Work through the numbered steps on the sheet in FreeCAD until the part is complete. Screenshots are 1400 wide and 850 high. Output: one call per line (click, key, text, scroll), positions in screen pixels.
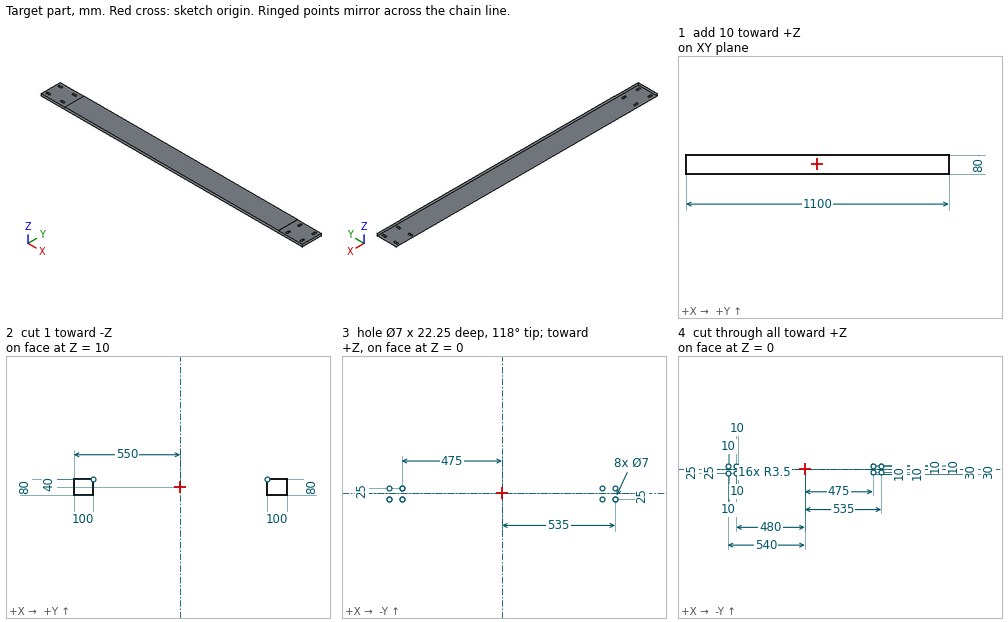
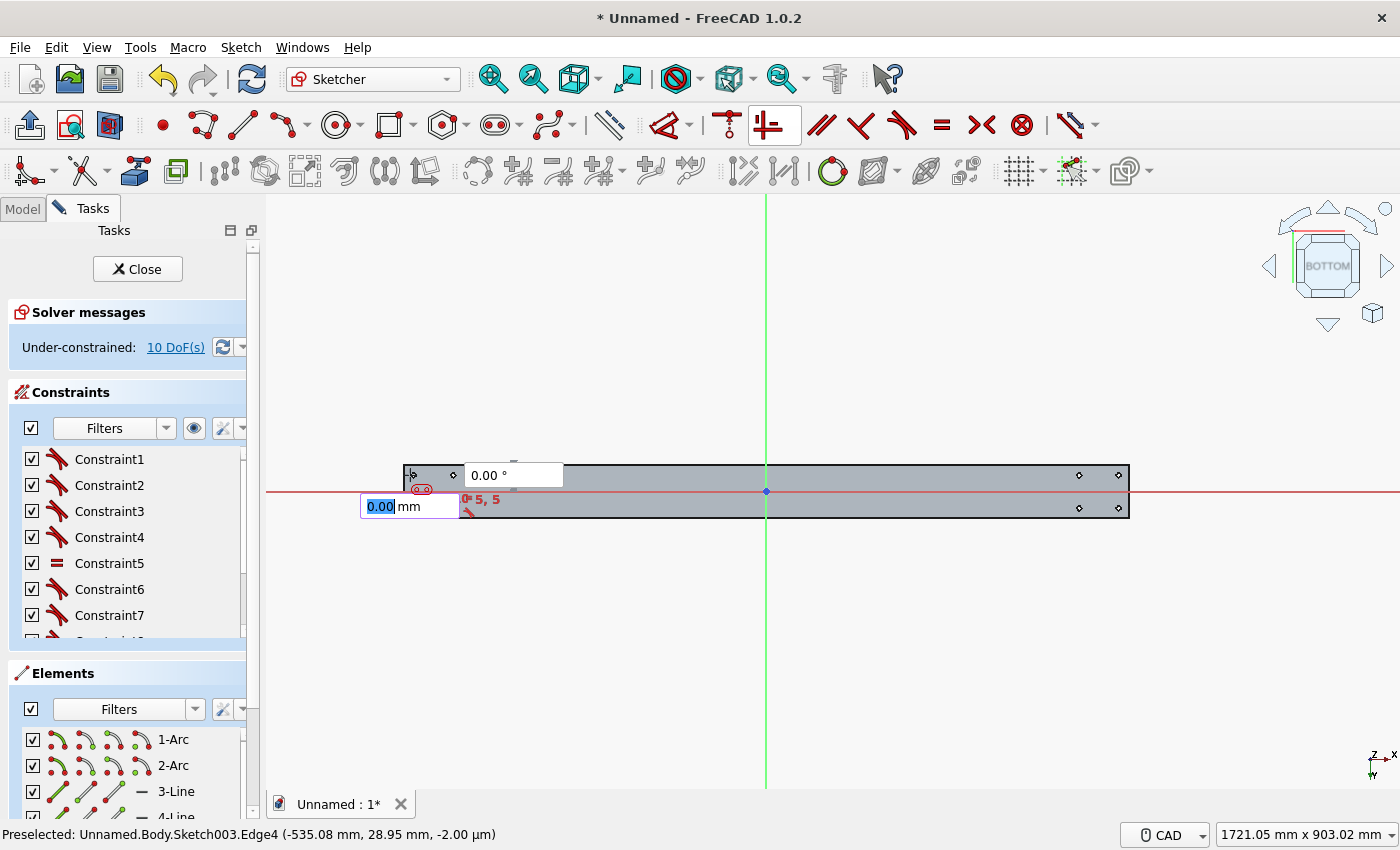
scroll(417, 475, up, 5)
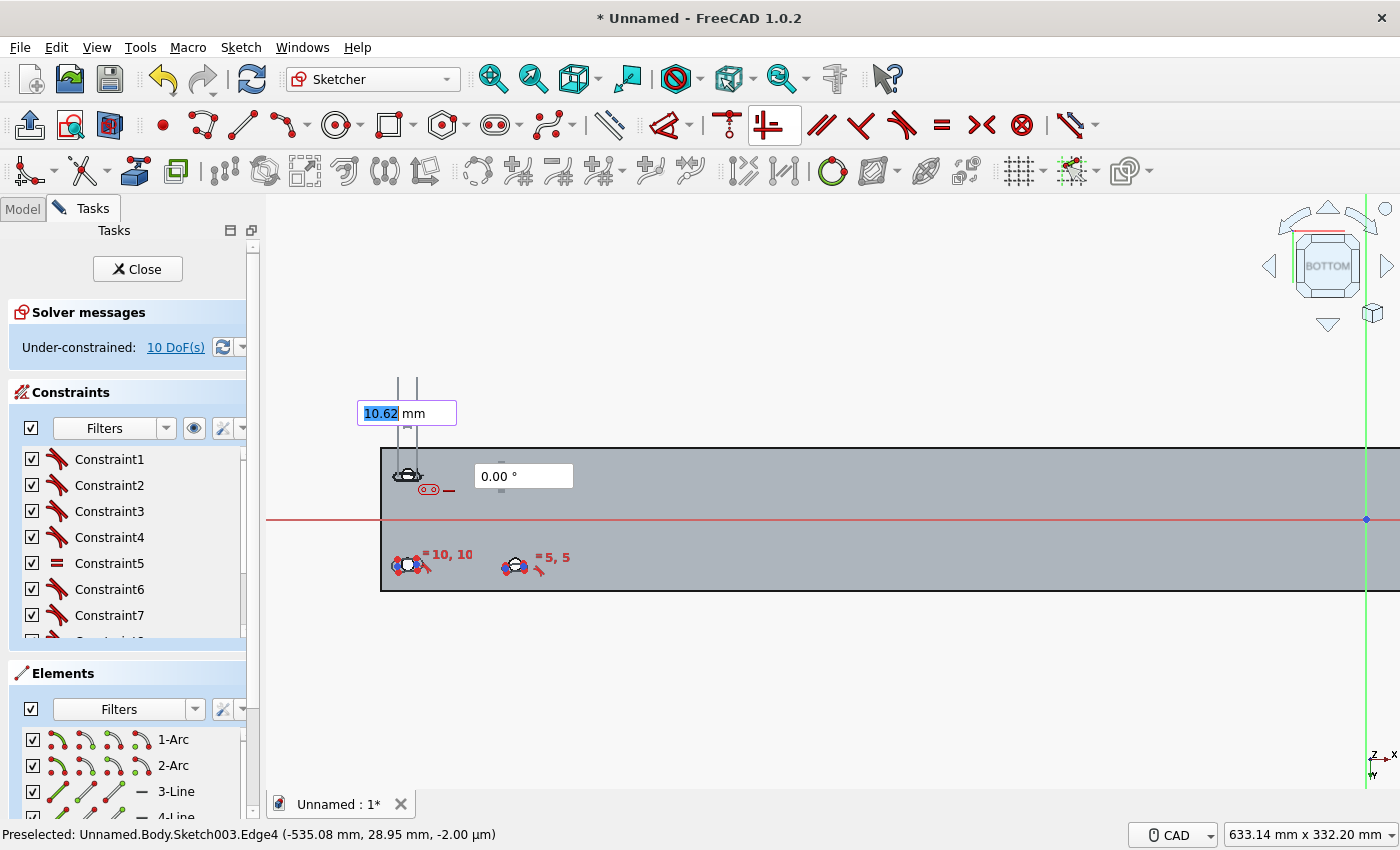
click(417, 474)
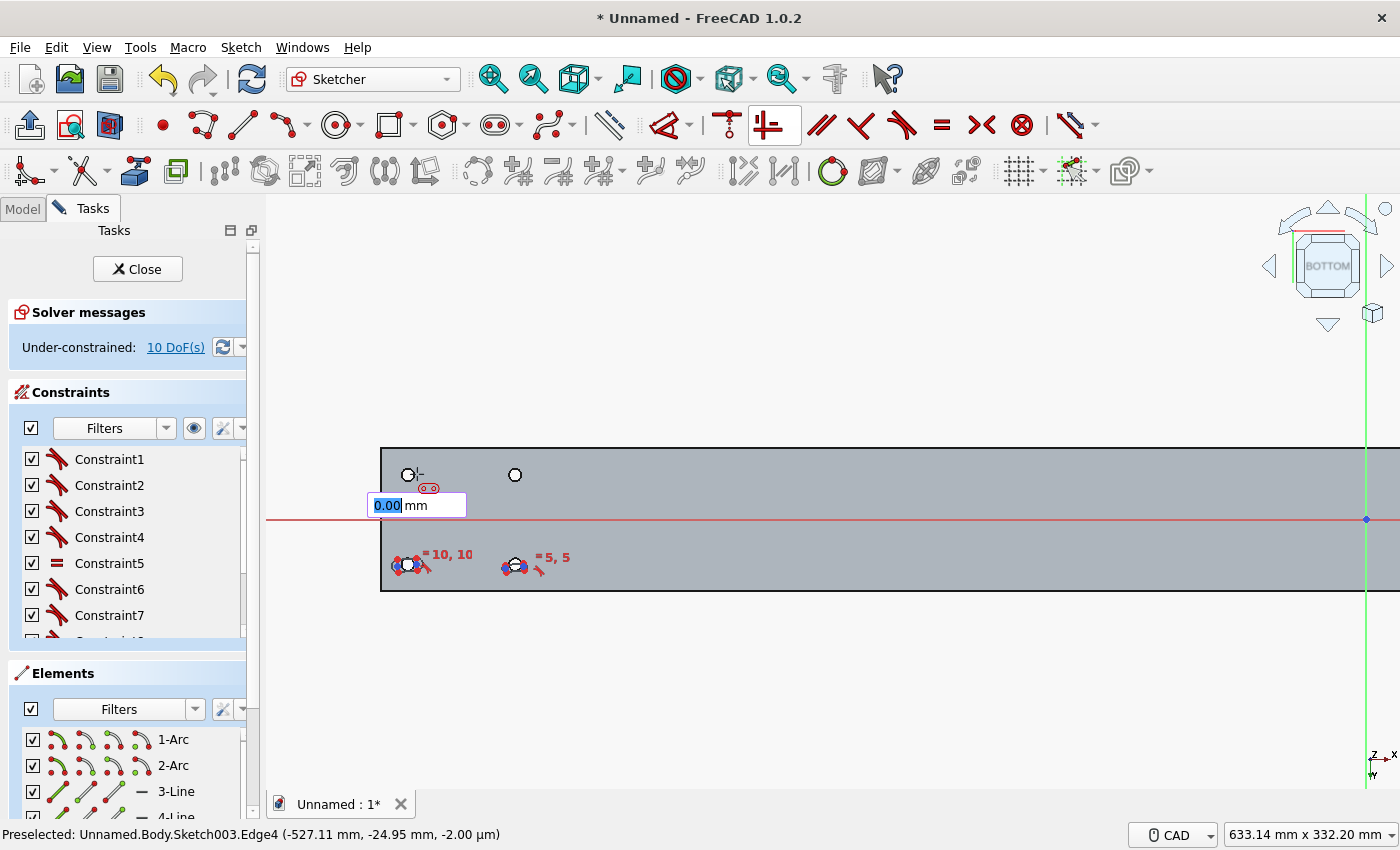
scroll(408, 481, up, 5)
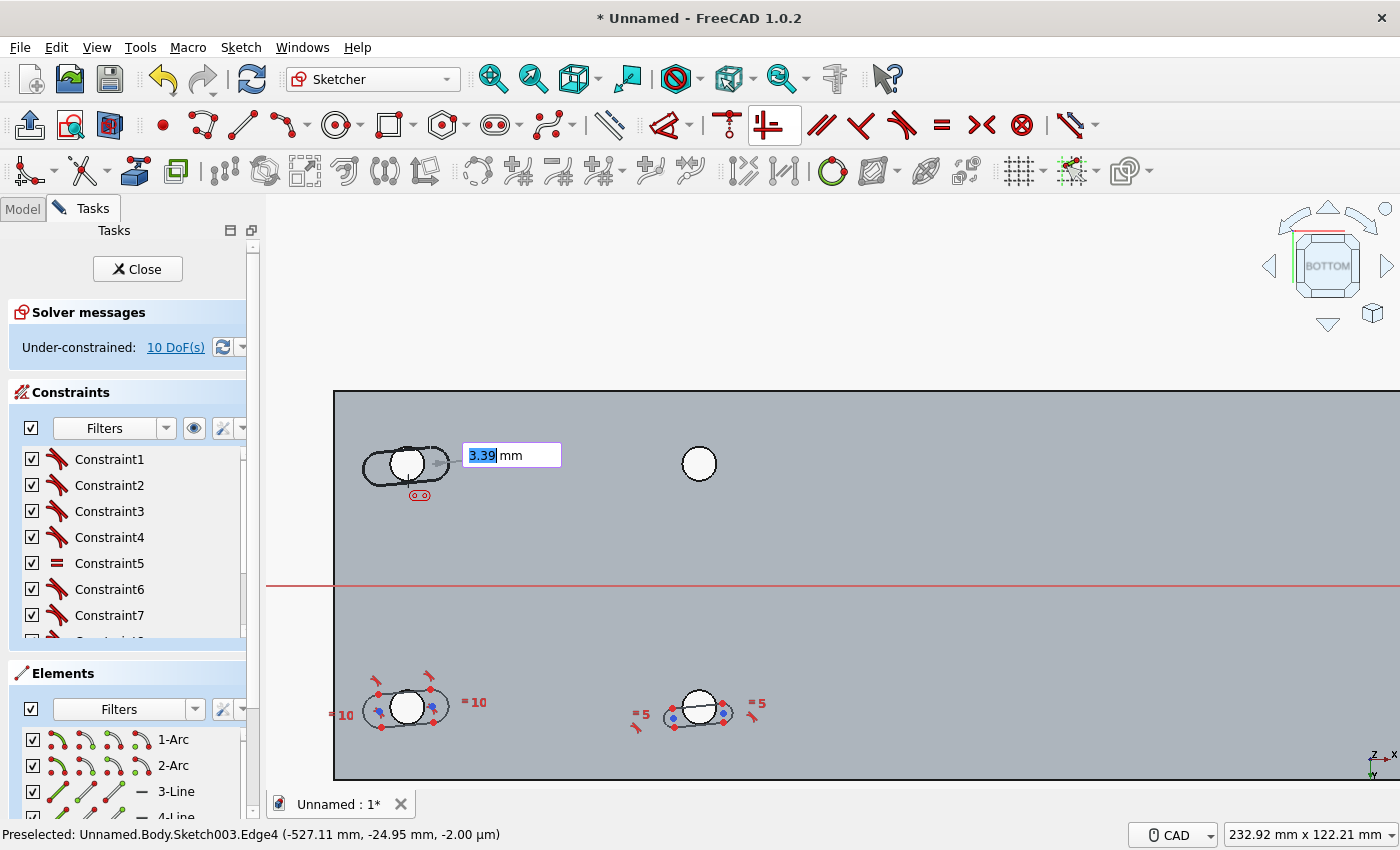
click(407, 481)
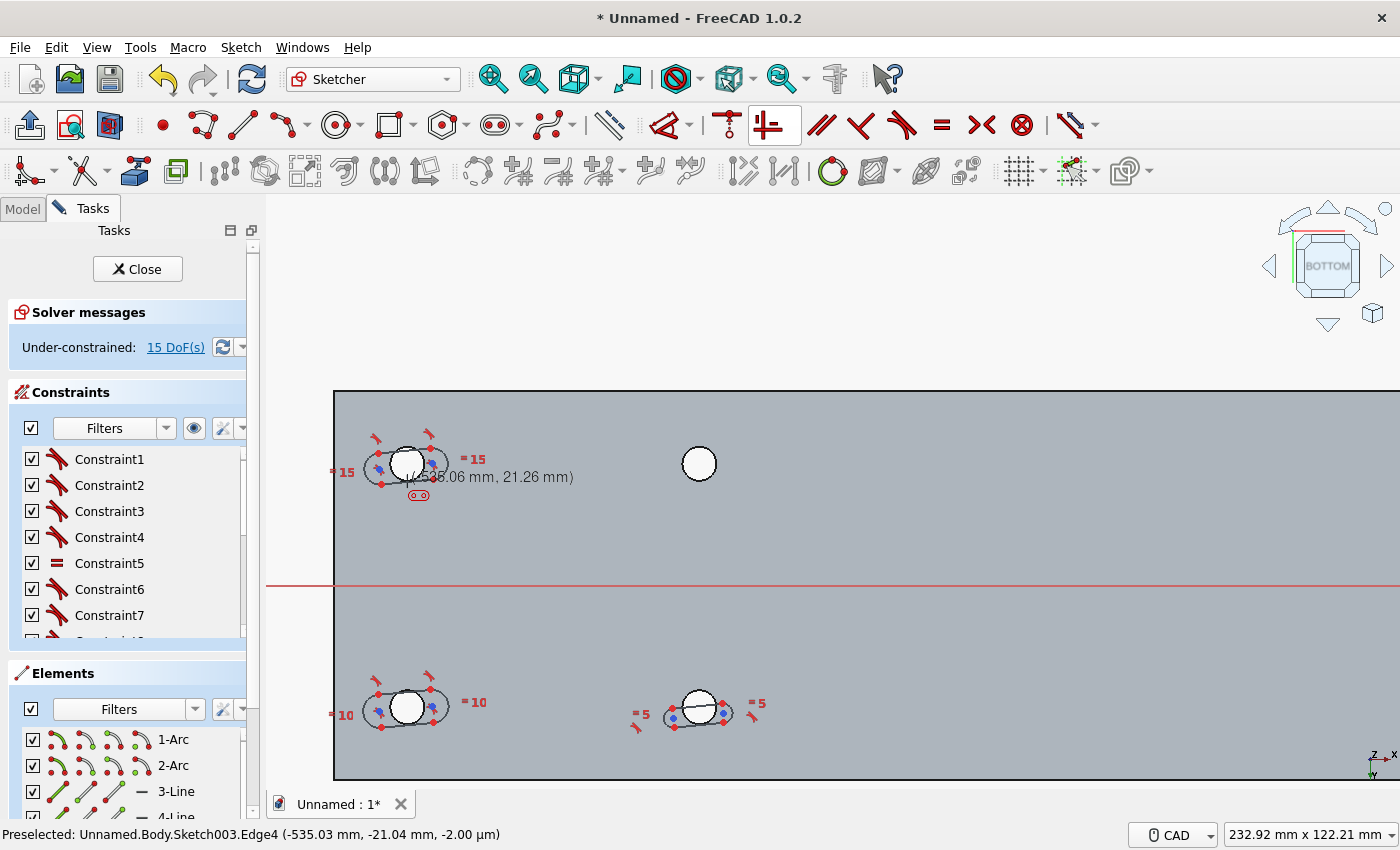
scroll(675, 464, up, 2)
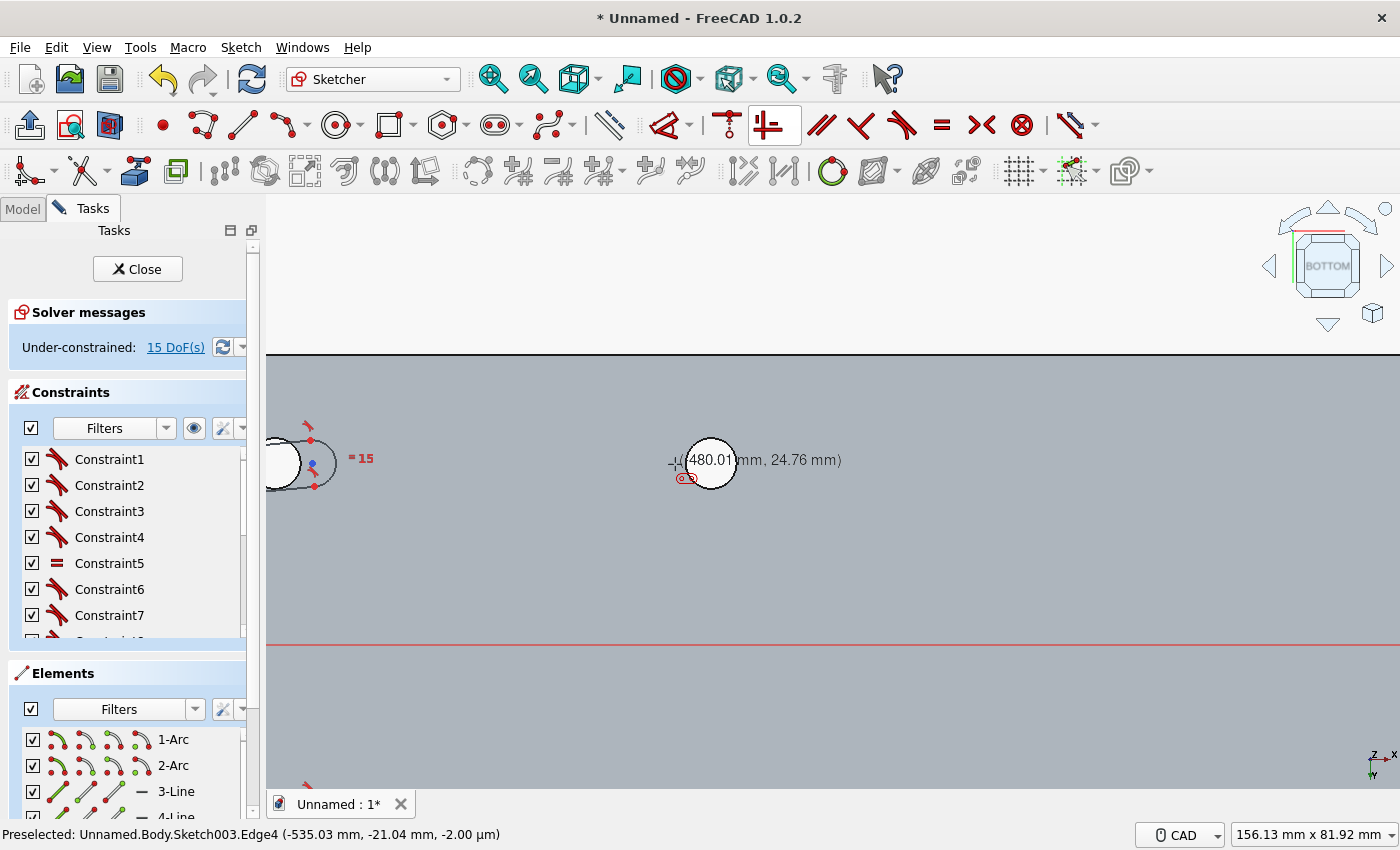
scroll(427, 476, down, 12)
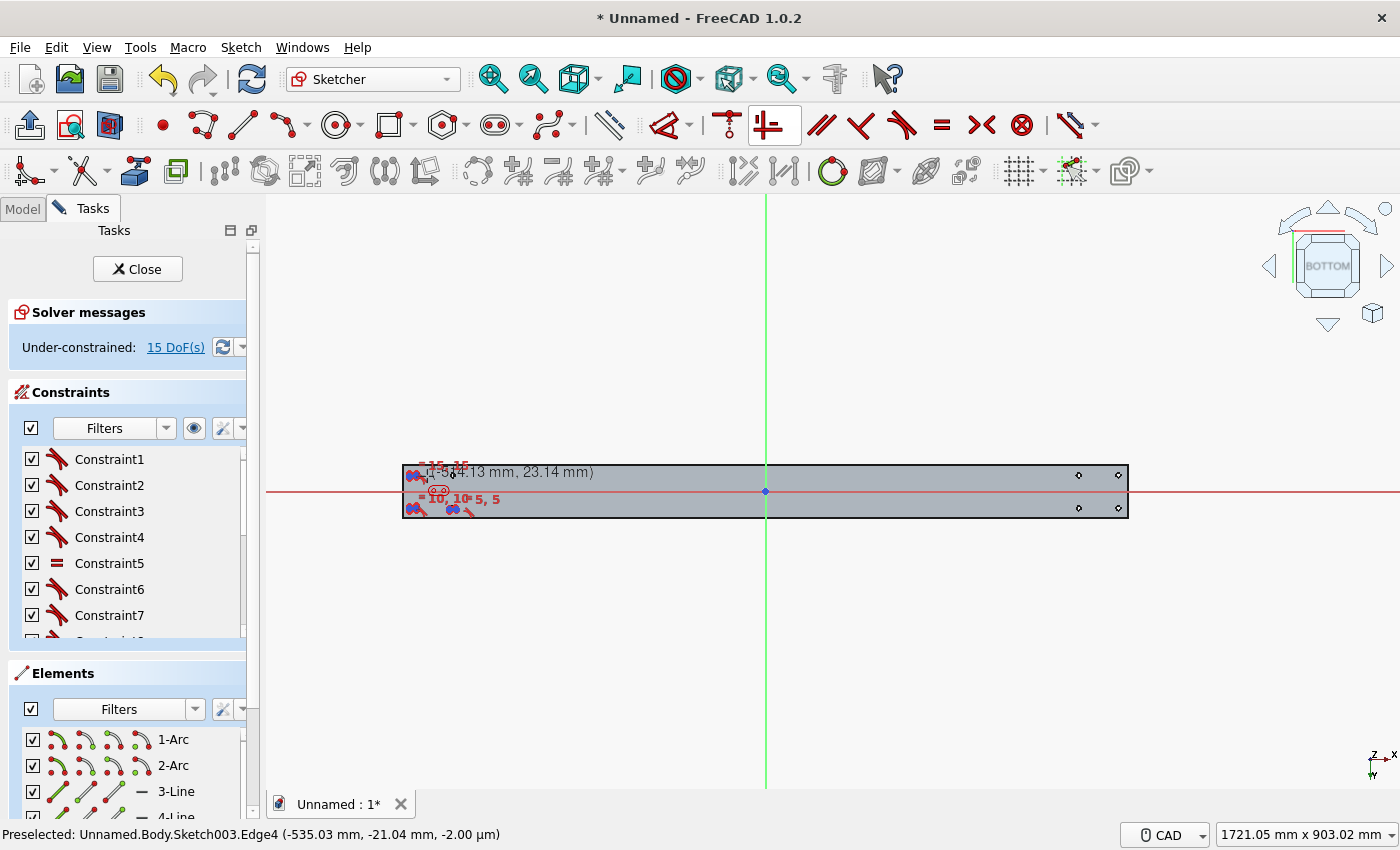
click(450, 475)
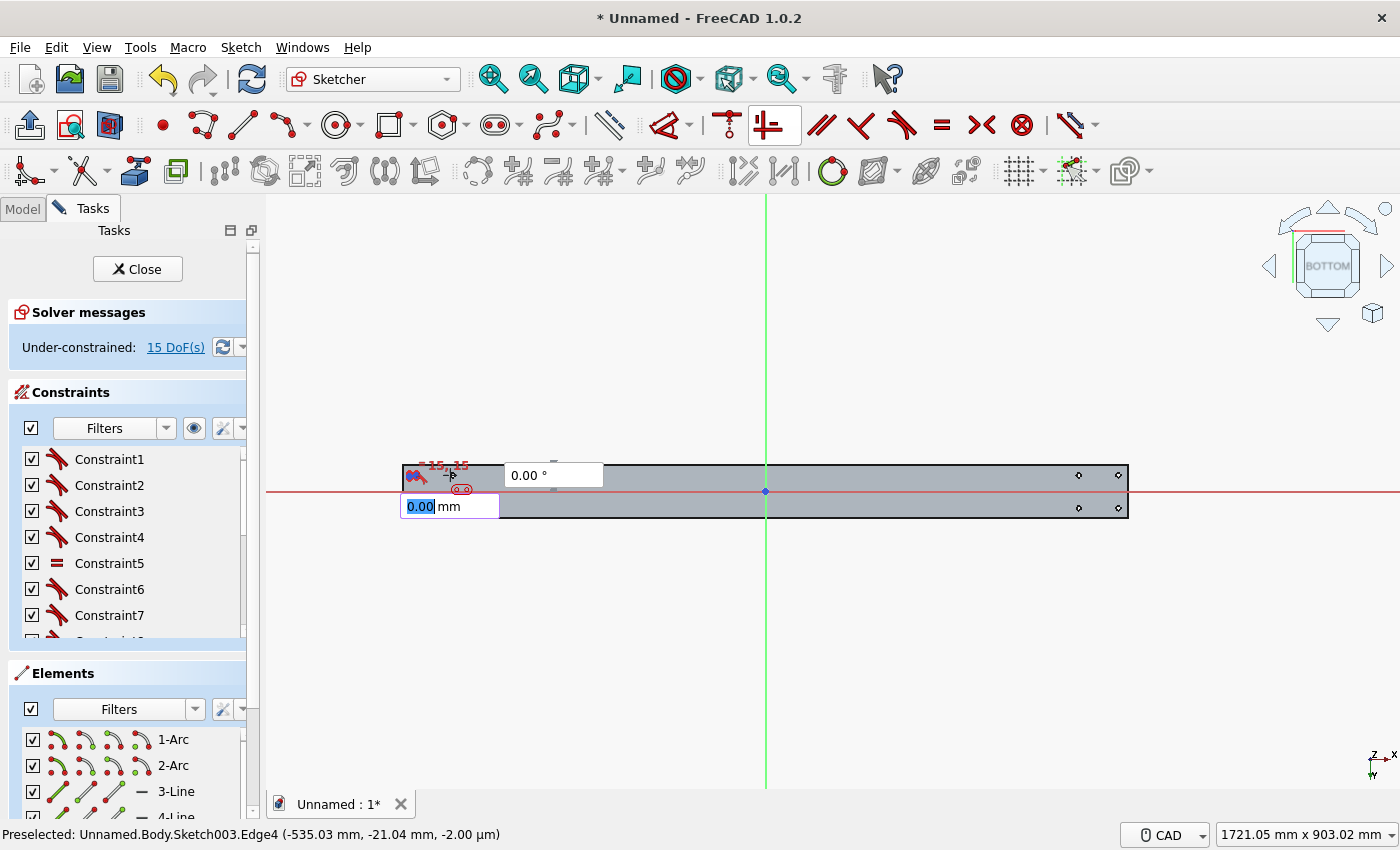
scroll(456, 475, up, 5)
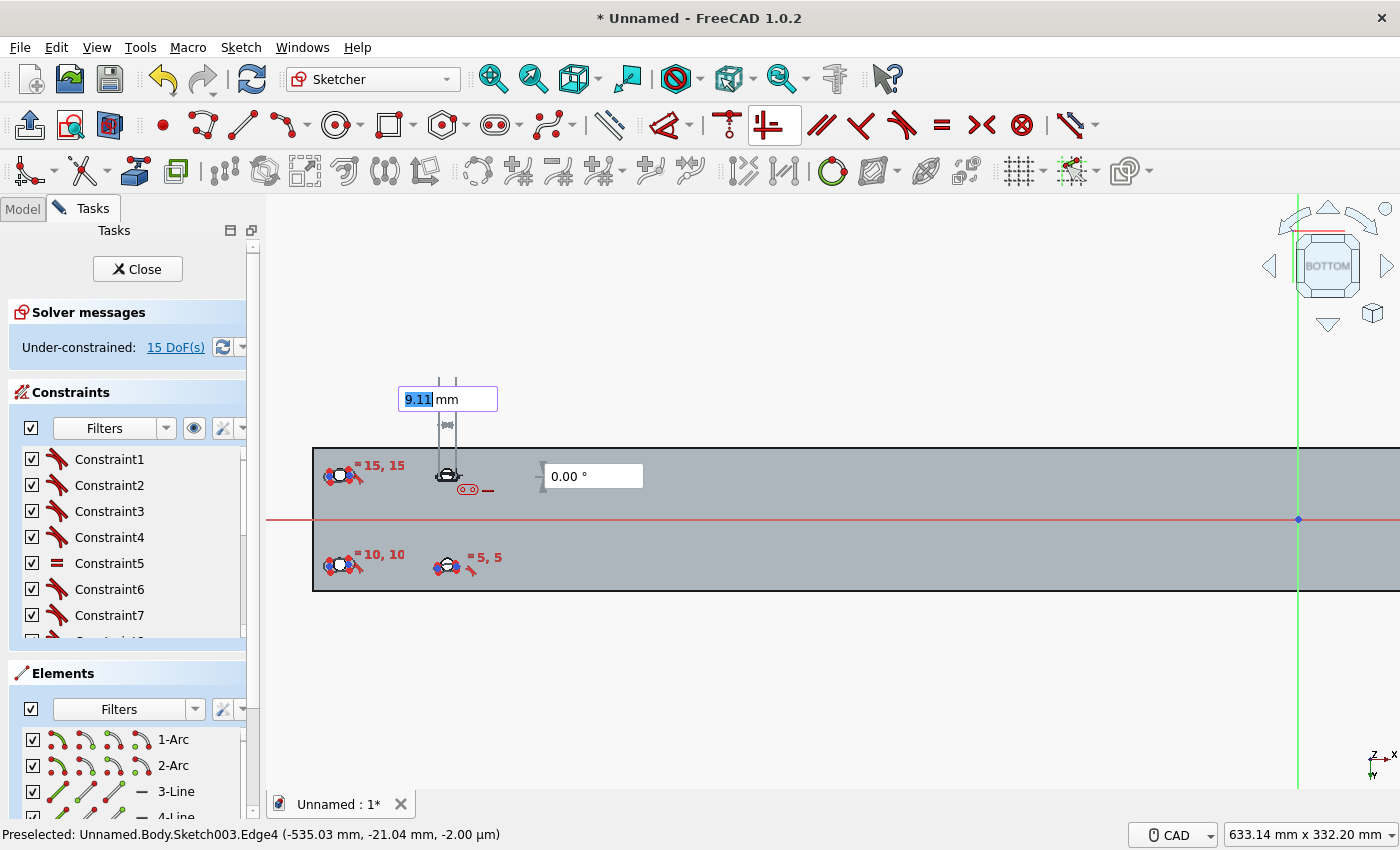
click(456, 474)